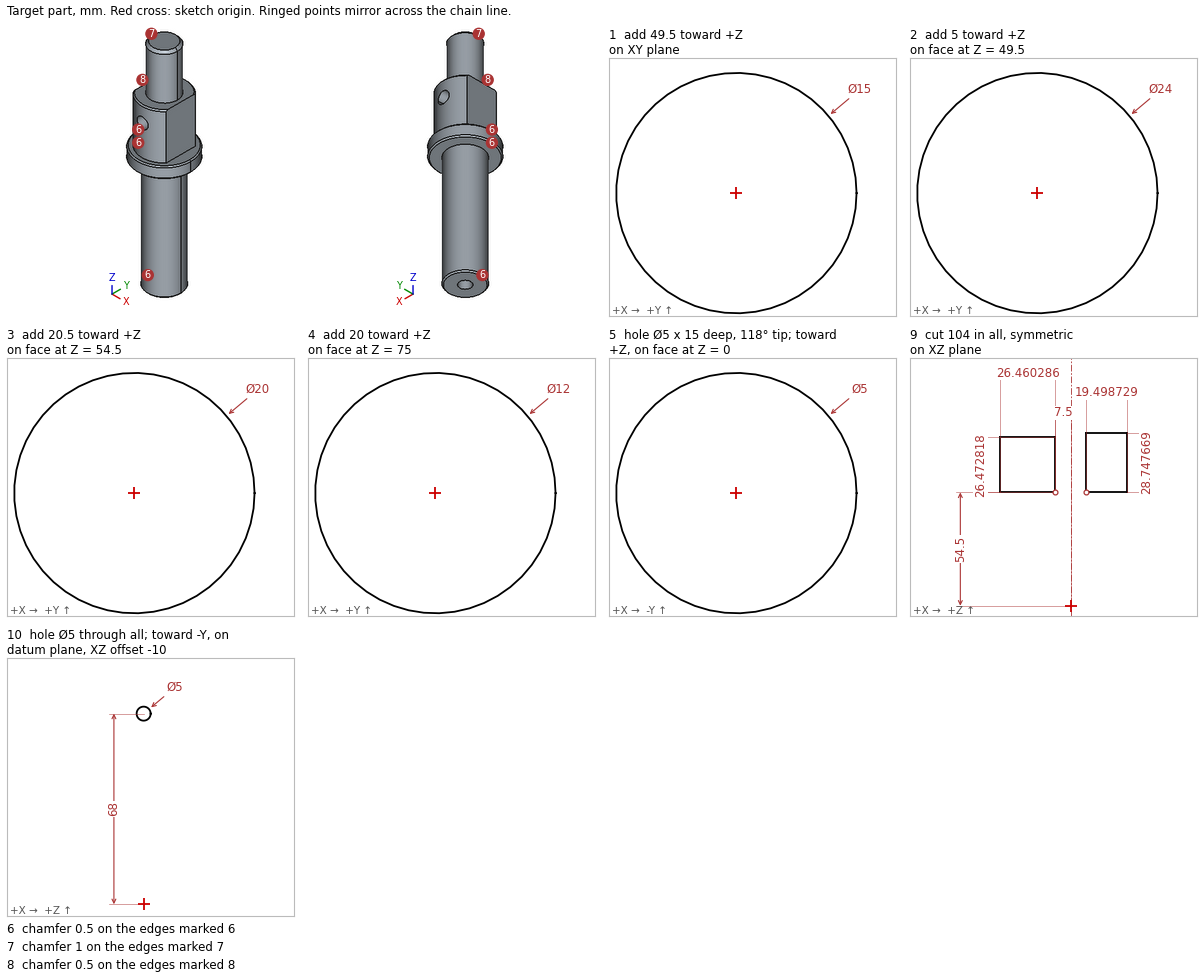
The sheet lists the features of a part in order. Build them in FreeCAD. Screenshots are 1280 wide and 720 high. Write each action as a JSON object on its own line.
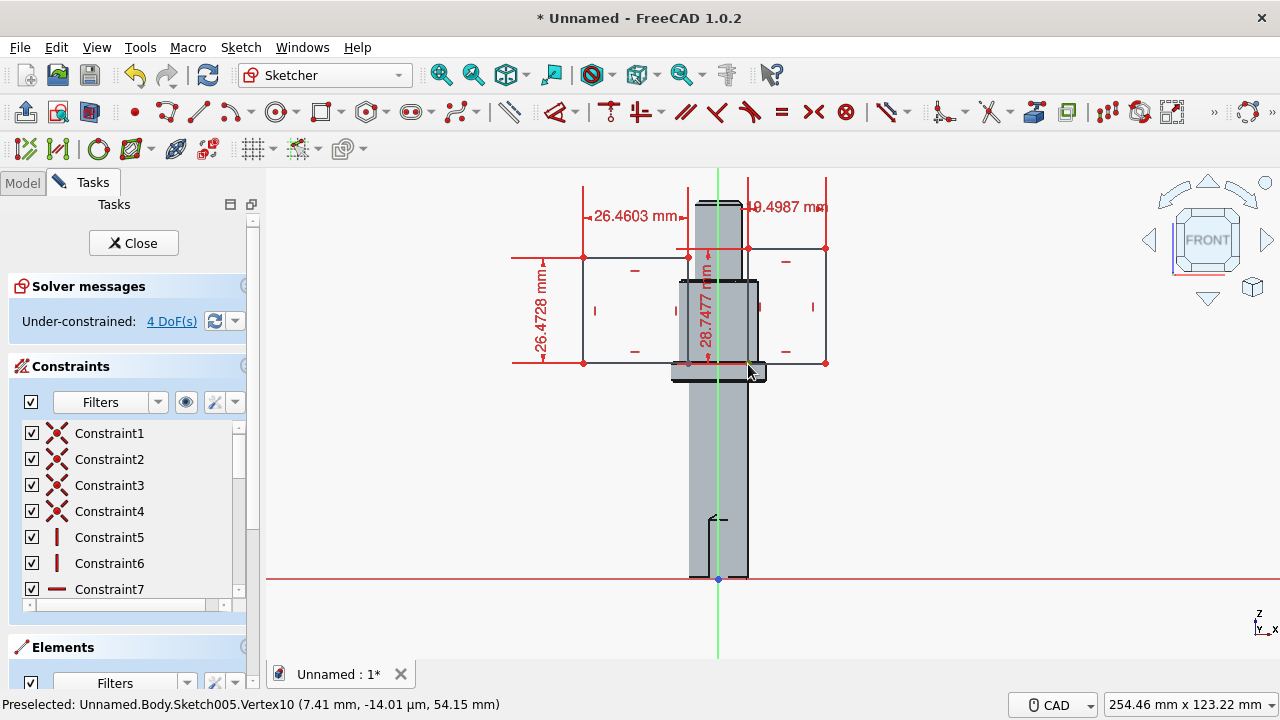
{"action": "left_click", "coordinate": [718, 538]}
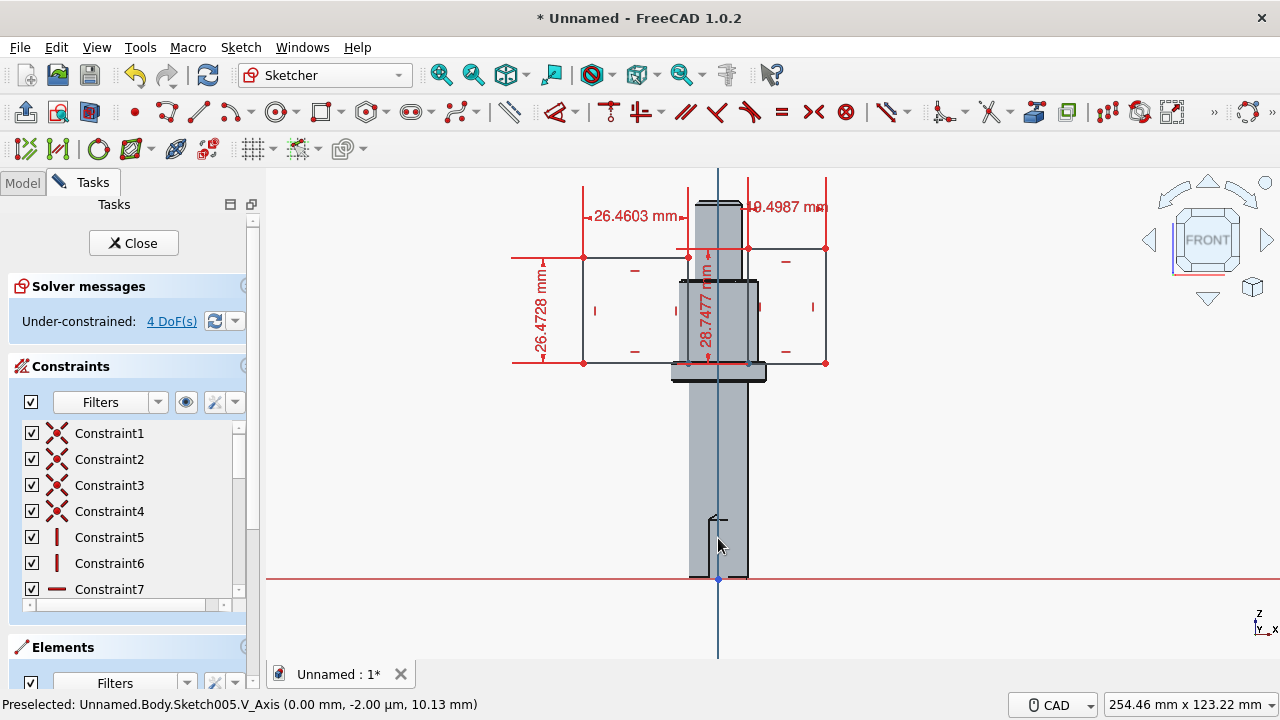
{"action": "key", "text": "s"}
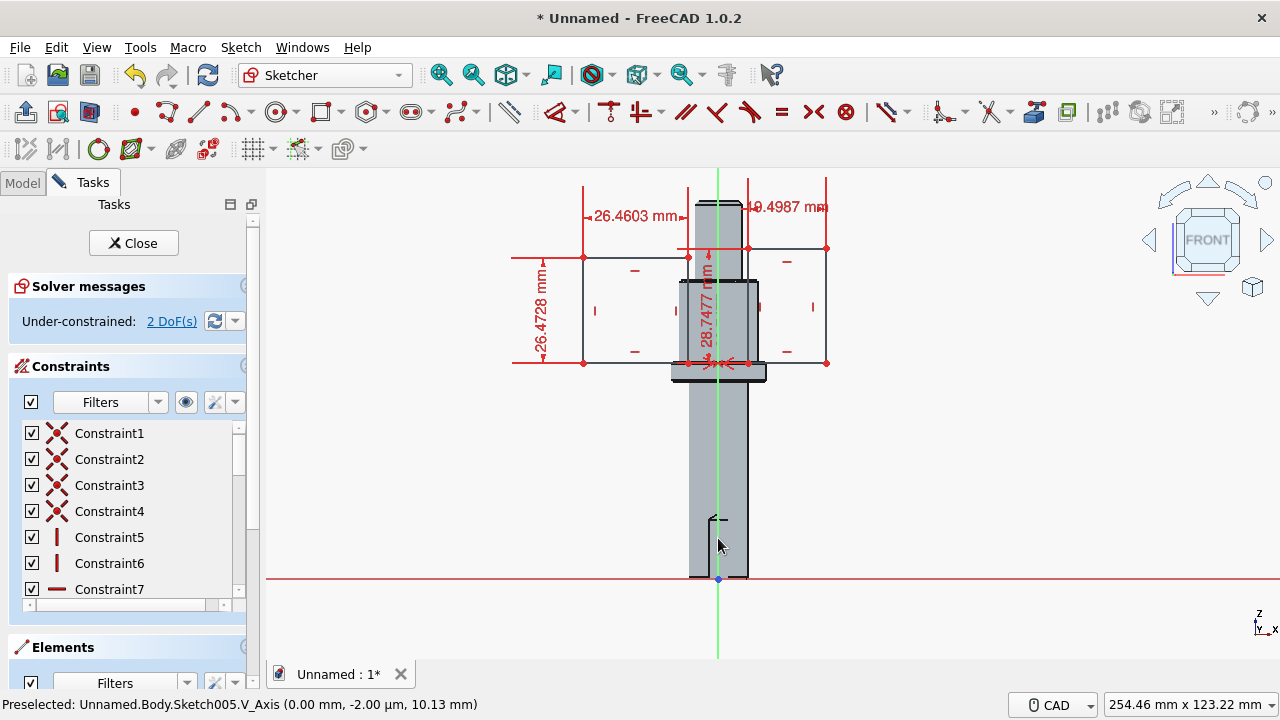
{"action": "key", "text": "d"}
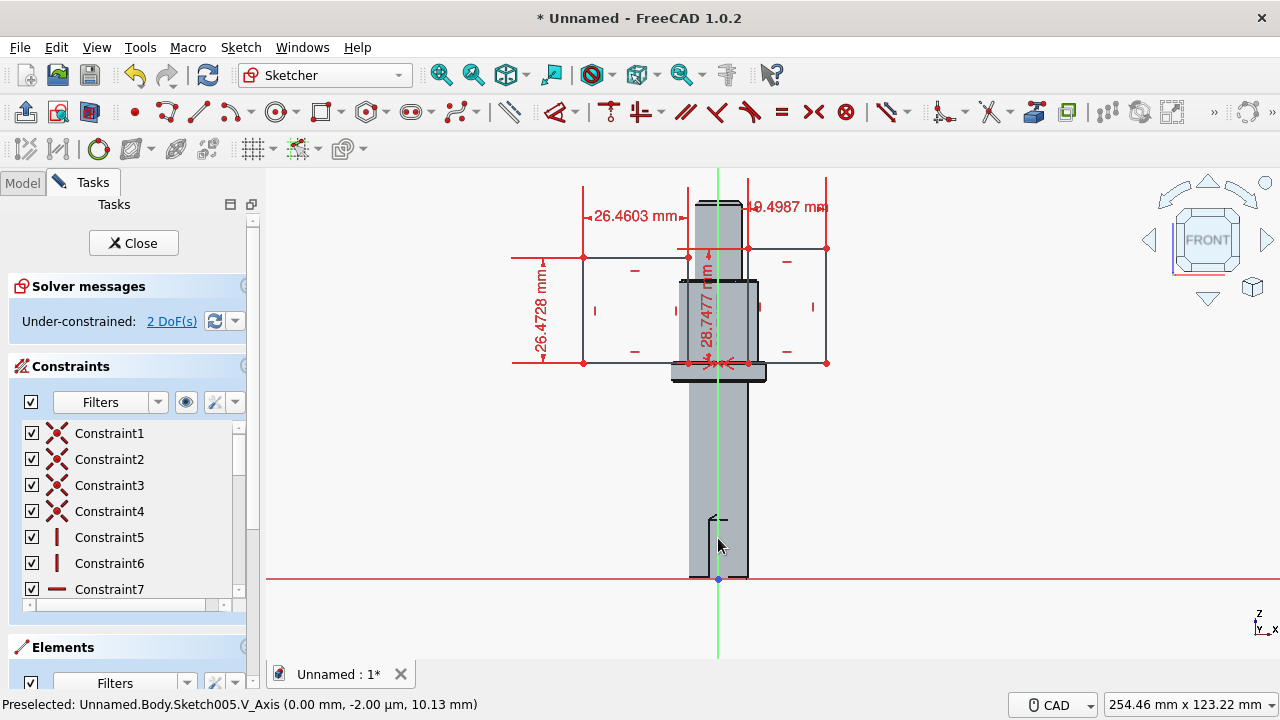
{"action": "scroll", "coordinate": [688, 363], "scroll_direction": "up", "scroll_amount": 2}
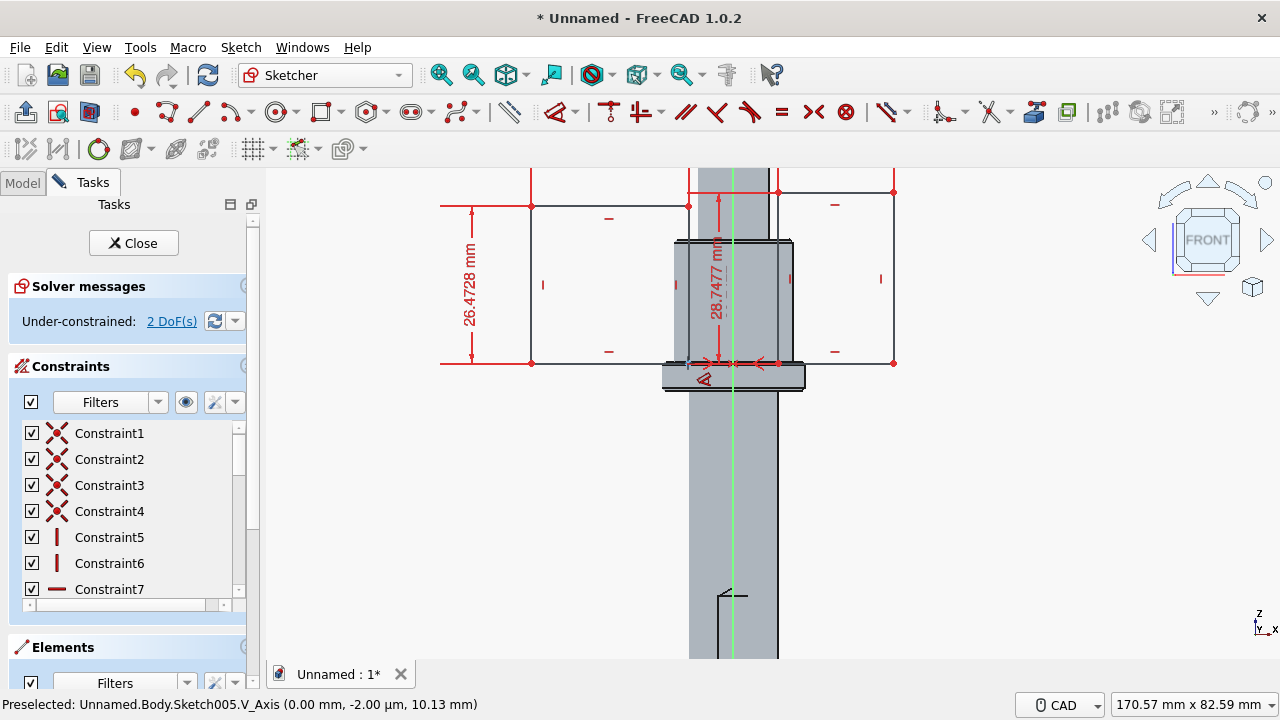
{"action": "left_click", "coordinate": [689, 364]}
{"action": "left_click", "coordinate": [711, 330]}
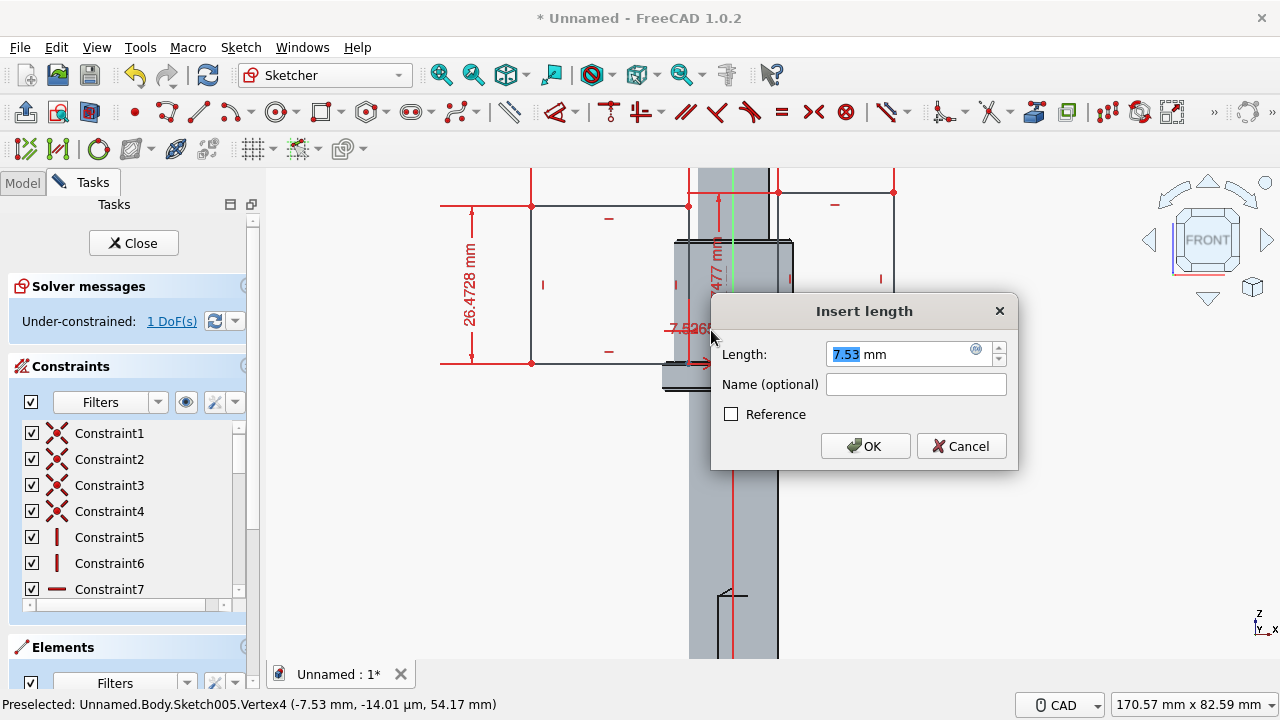
{"action": "type", "text": "7.5"}
{"action": "key", "text": "Return"}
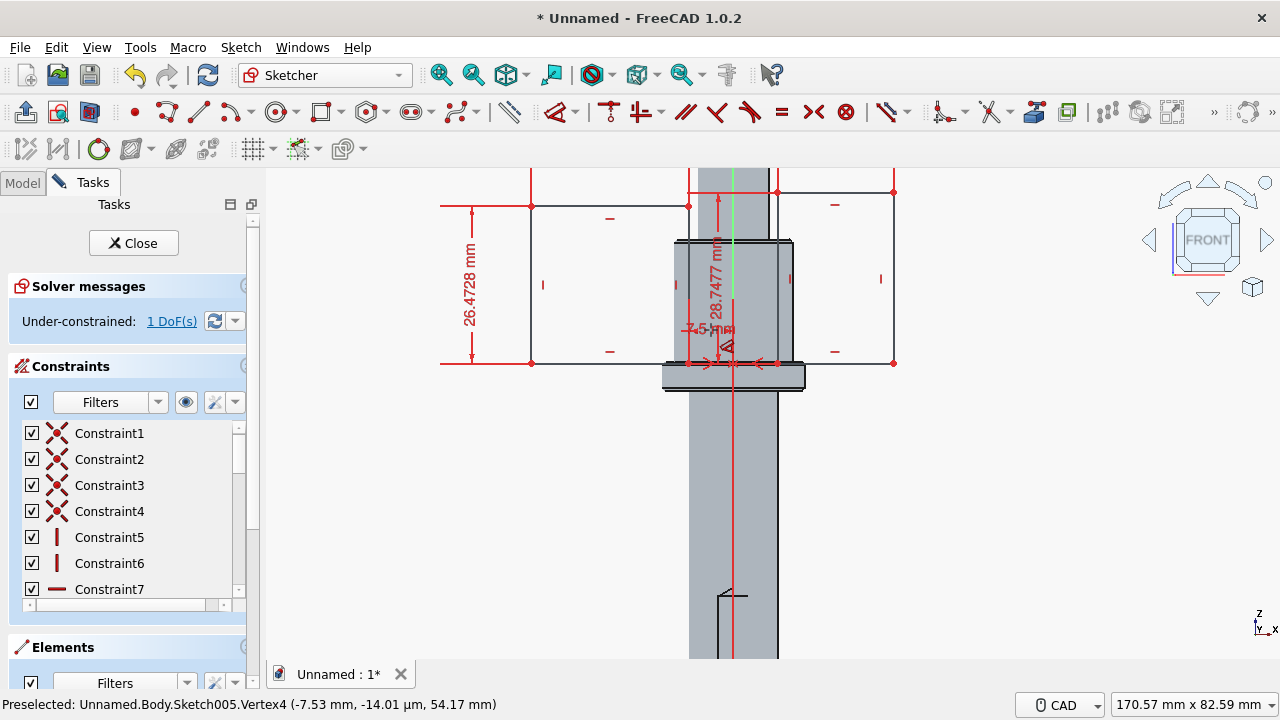
{"action": "left_click", "coordinate": [531, 364]}
{"action": "left_click", "coordinate": [497, 497]}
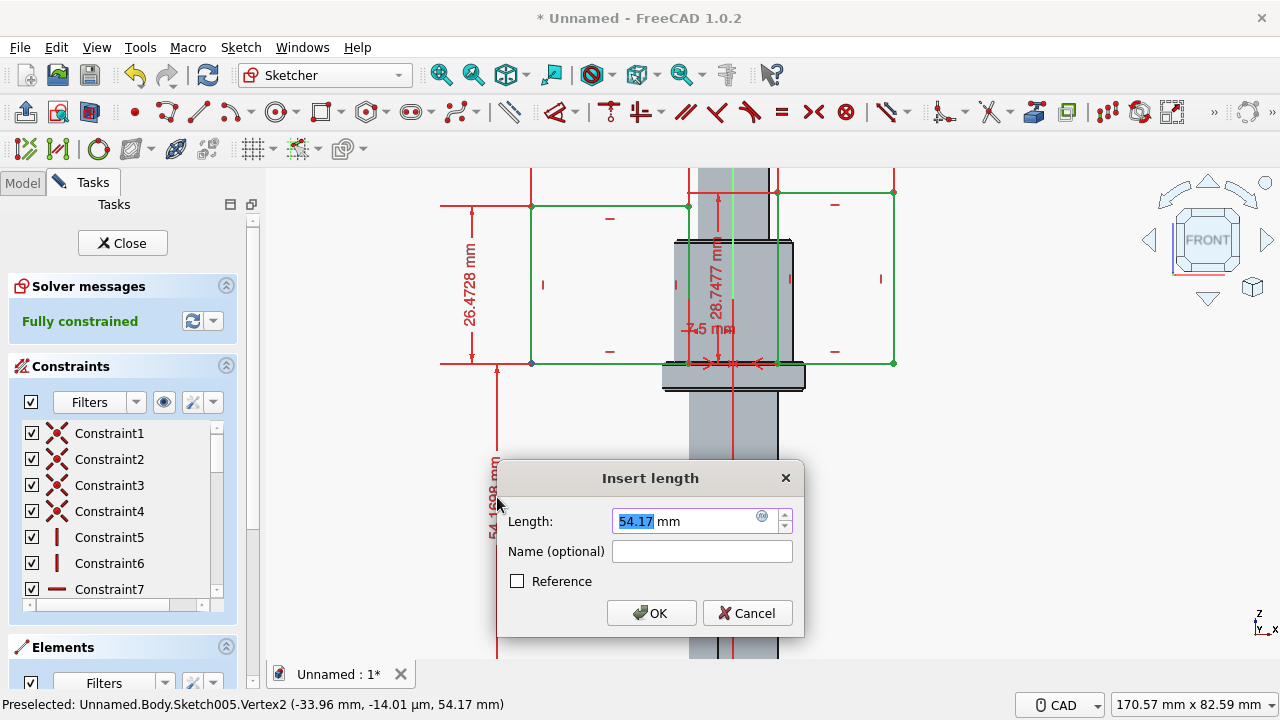
{"action": "type", "text": "54.5"}
{"action": "key", "text": "Return"}
{"action": "key", "text": "Escape"}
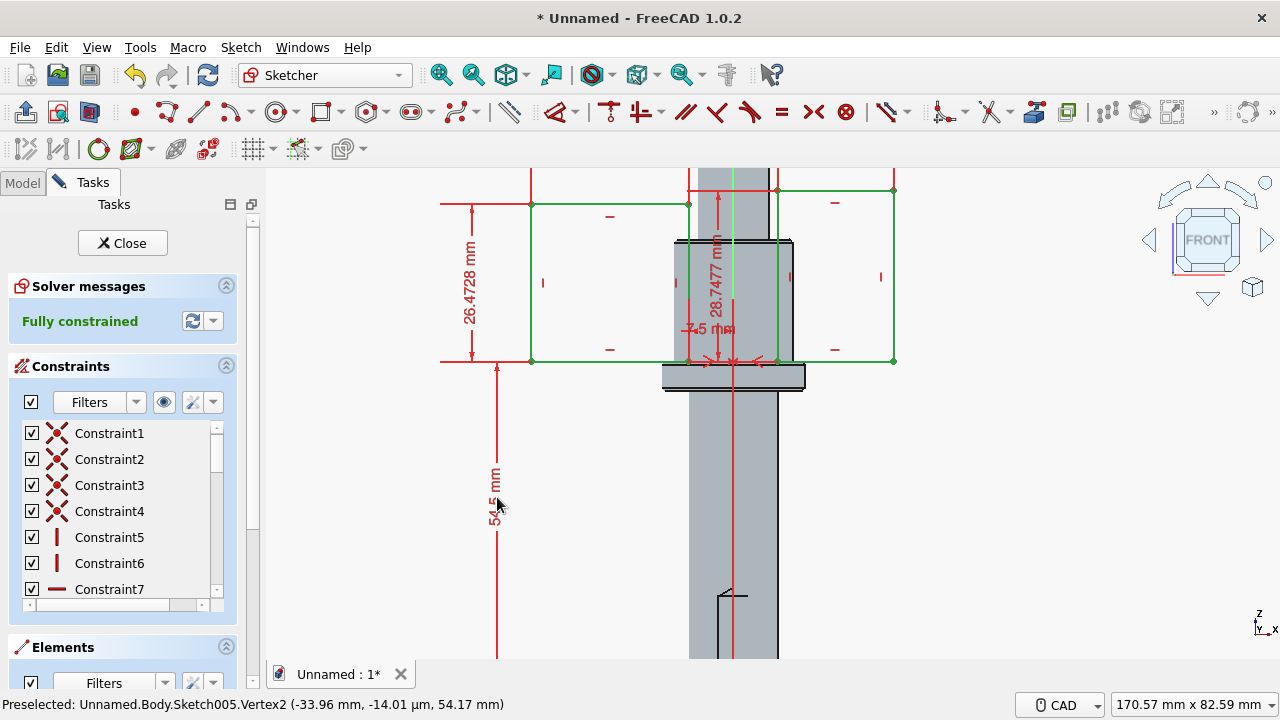
{"action": "left_click", "coordinate": [123, 243]}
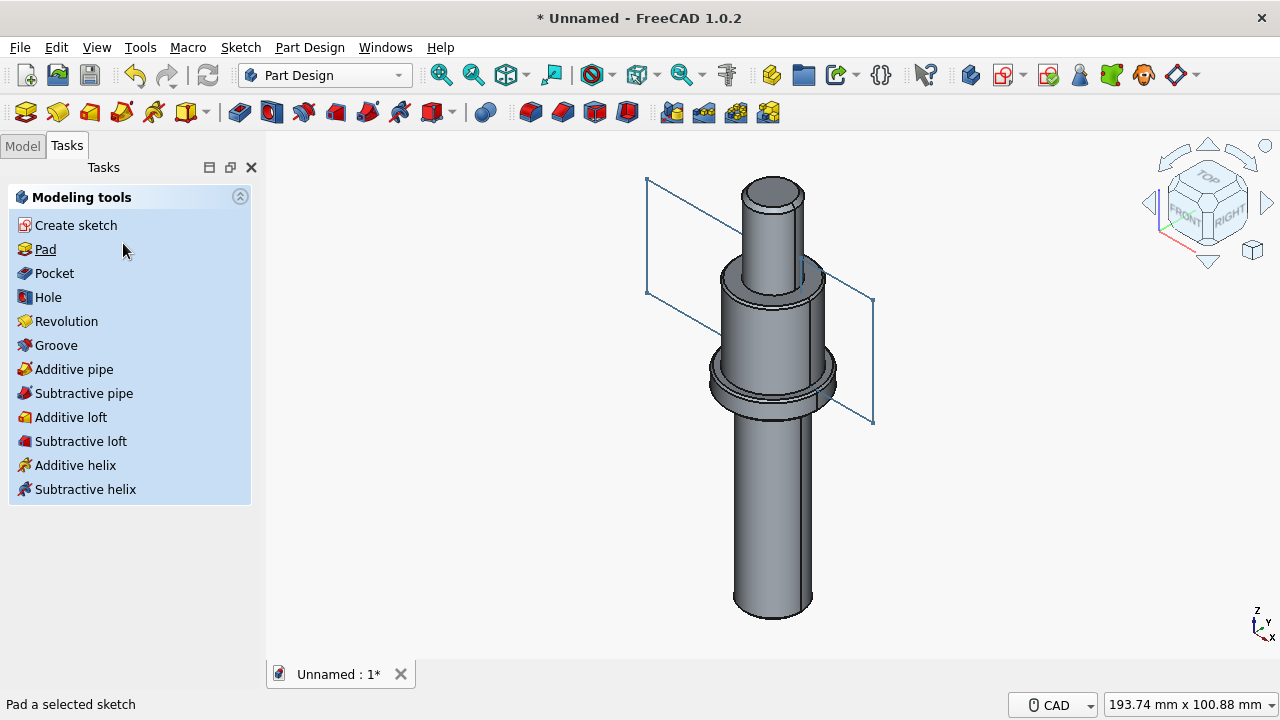
{"action": "left_click", "coordinate": [240, 112]}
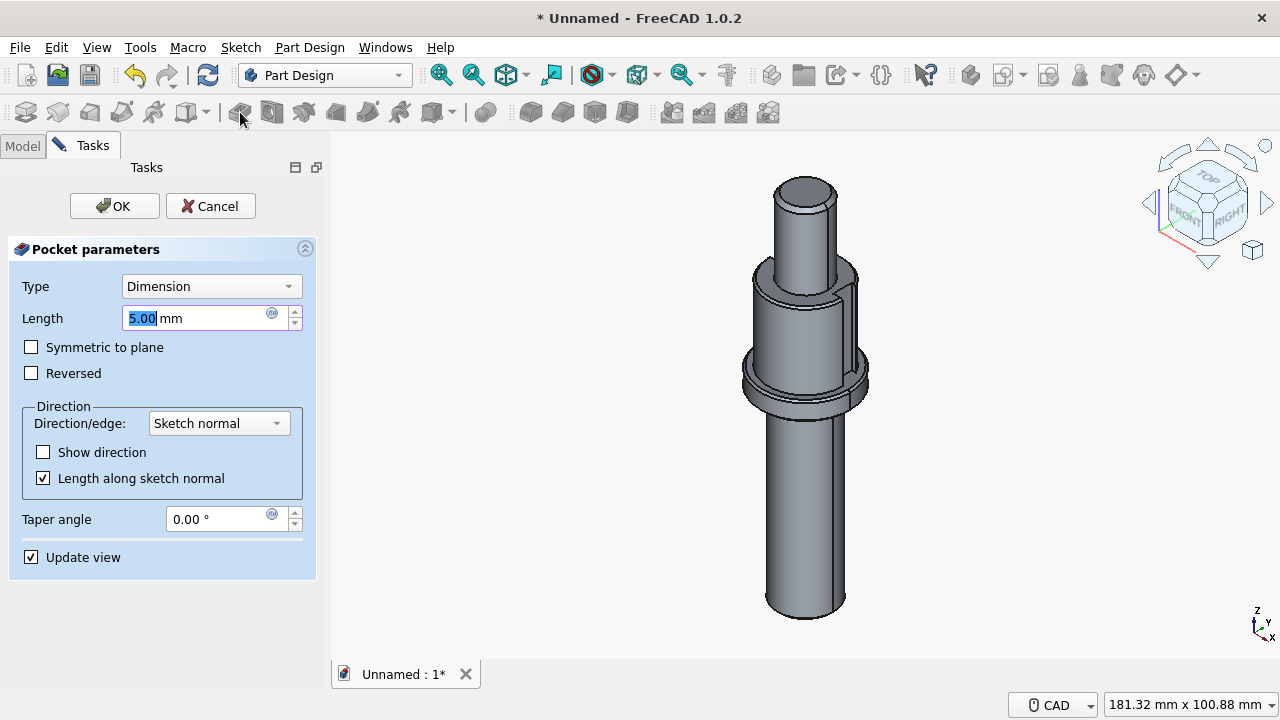
{"action": "type", "text": "104"}
{"action": "key", "text": "Tab"}